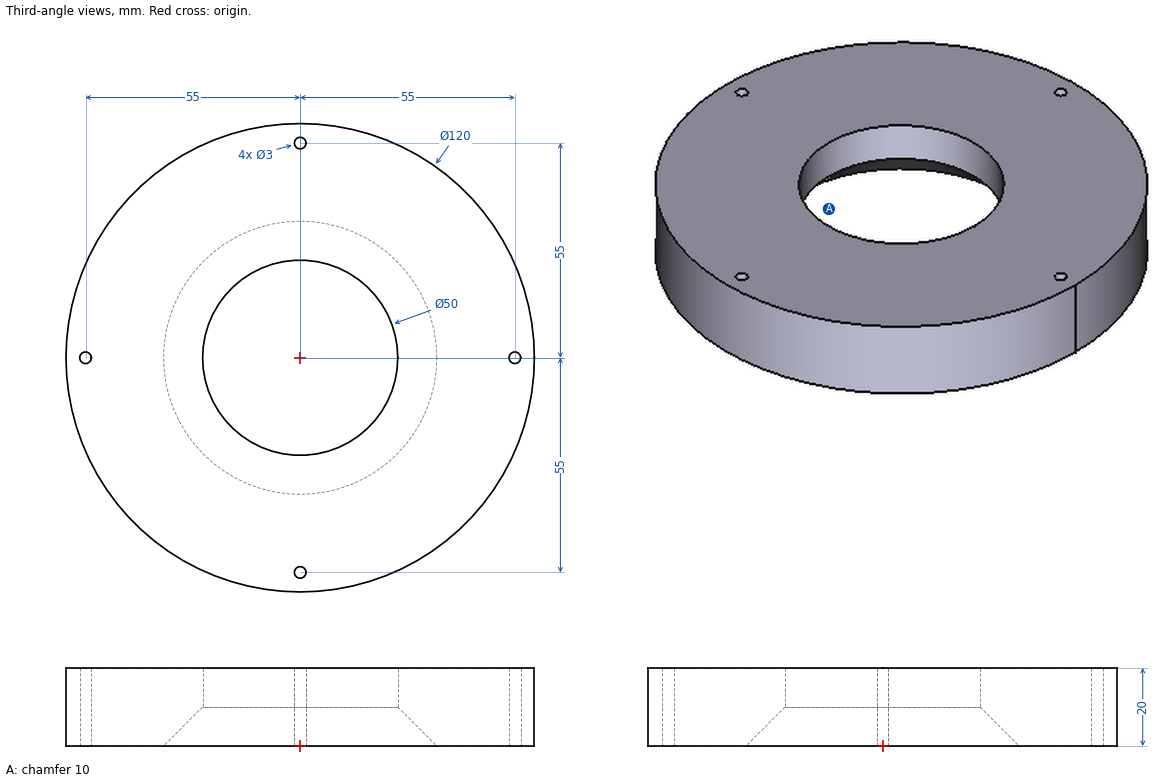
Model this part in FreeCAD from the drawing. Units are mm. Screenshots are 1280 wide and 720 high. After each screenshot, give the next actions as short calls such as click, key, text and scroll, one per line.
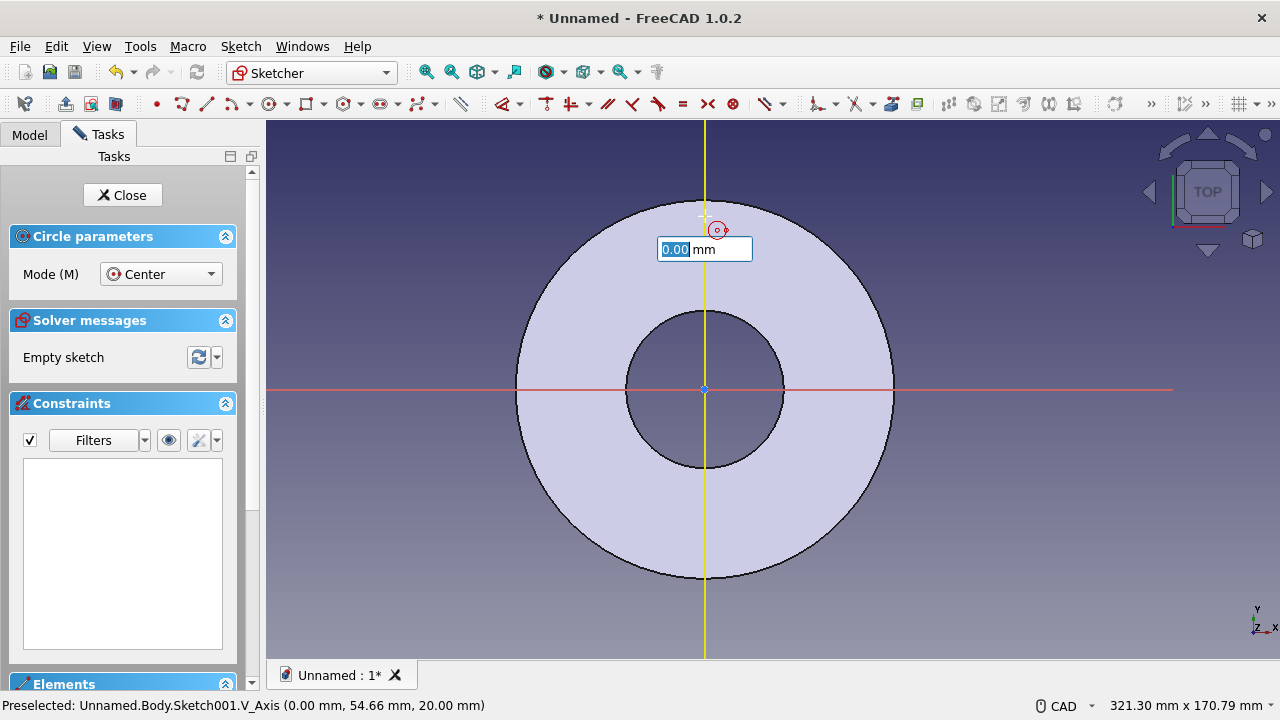
scroll(709, 214, up, 7)
move(709, 215)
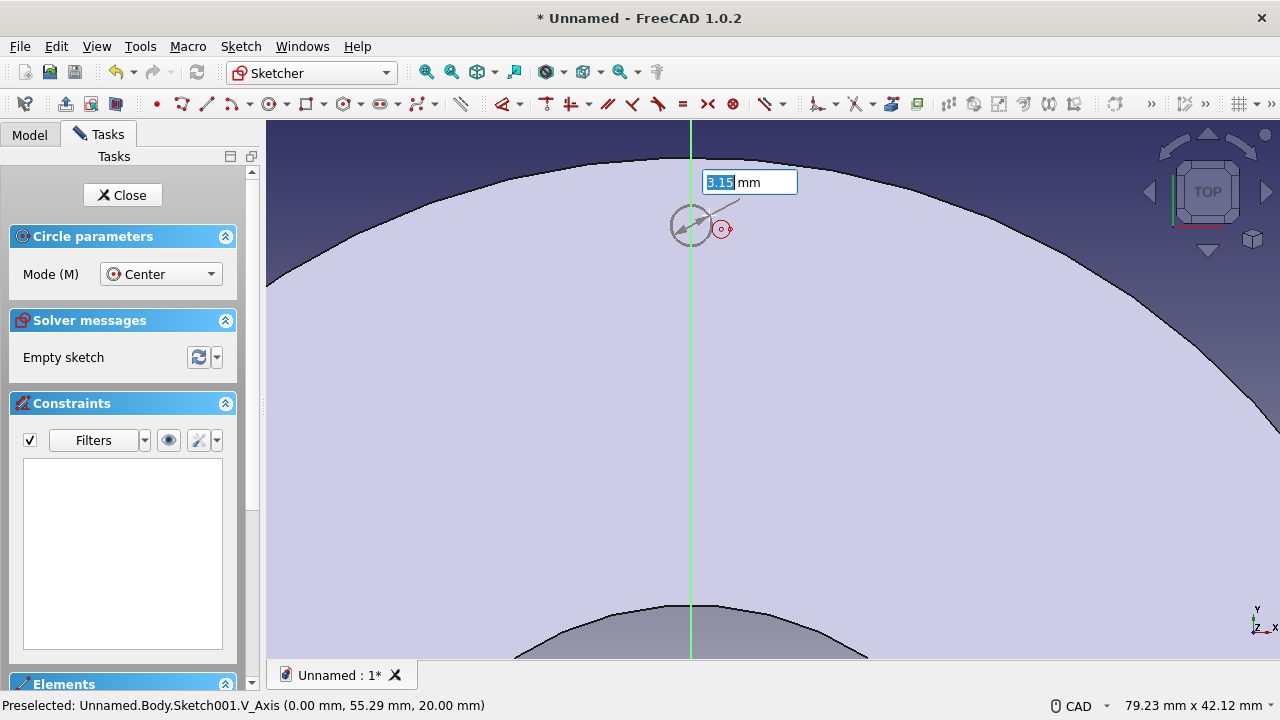
text(3)
key(Return)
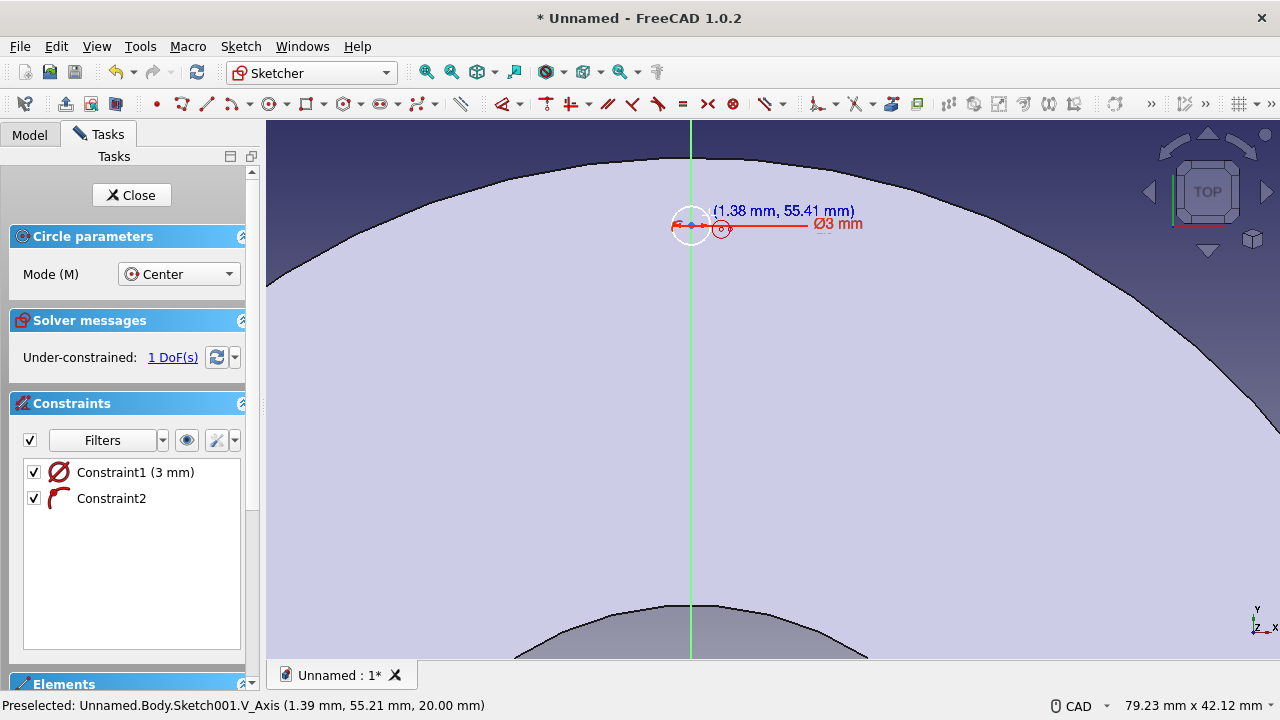
scroll(709, 214, down, 7)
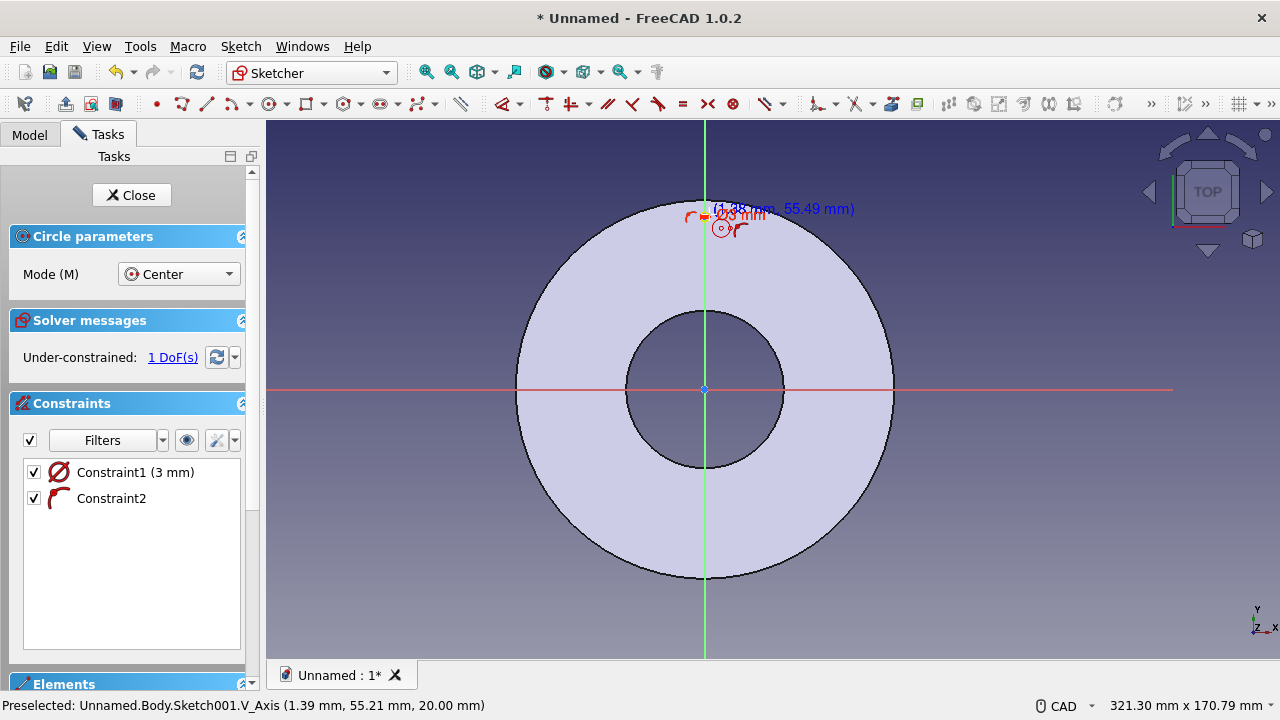
scroll(879, 389, up, 8)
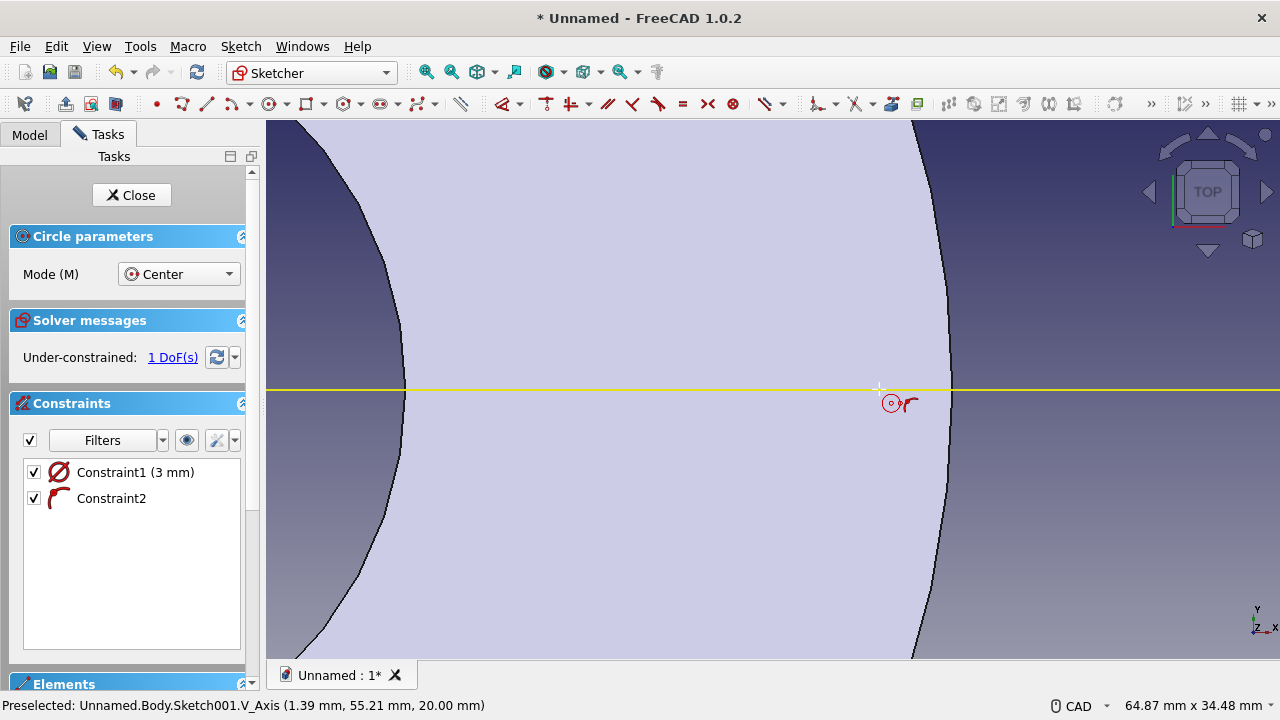
scroll(879, 390, down, 8)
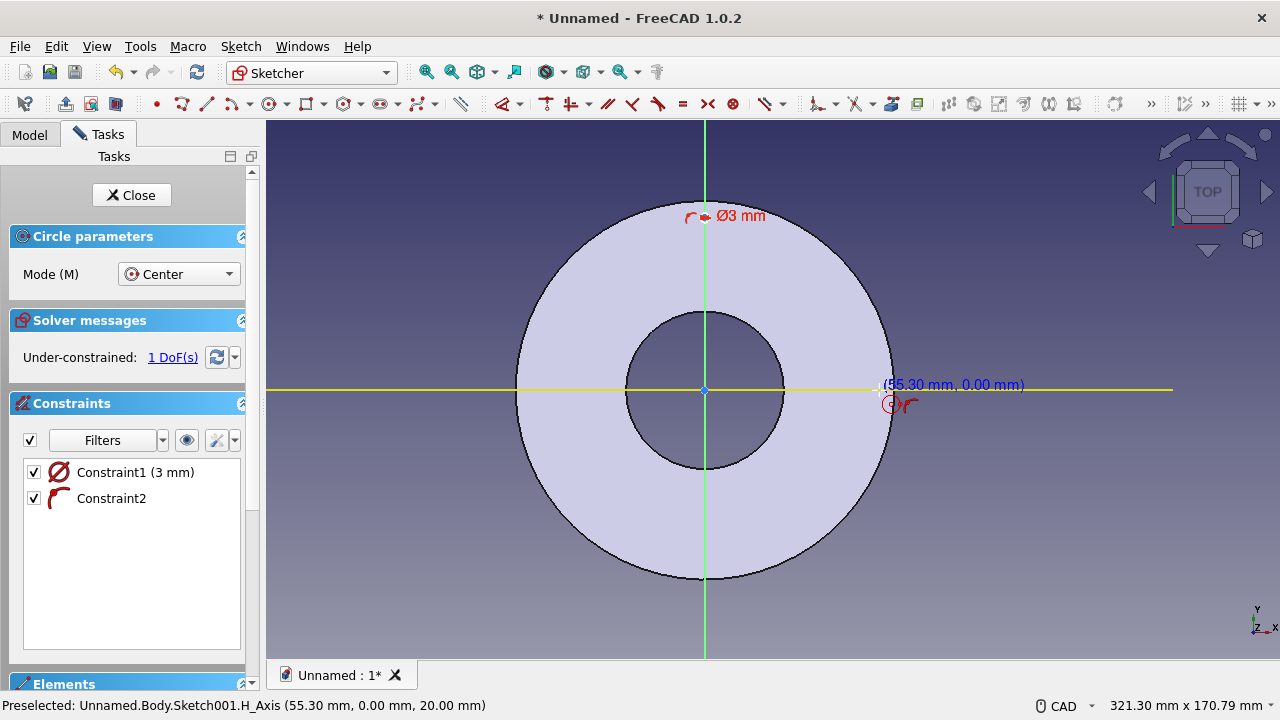
click(879, 390)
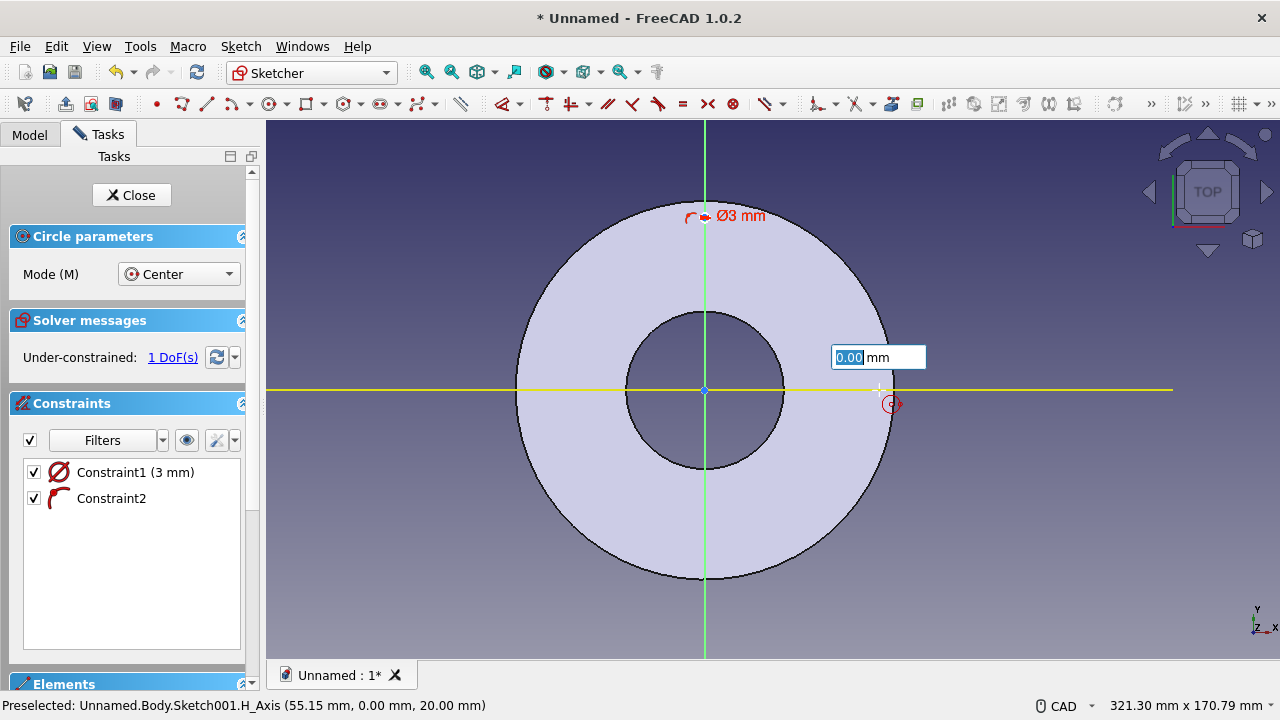
scroll(877, 395, up, 7)
move(875, 392)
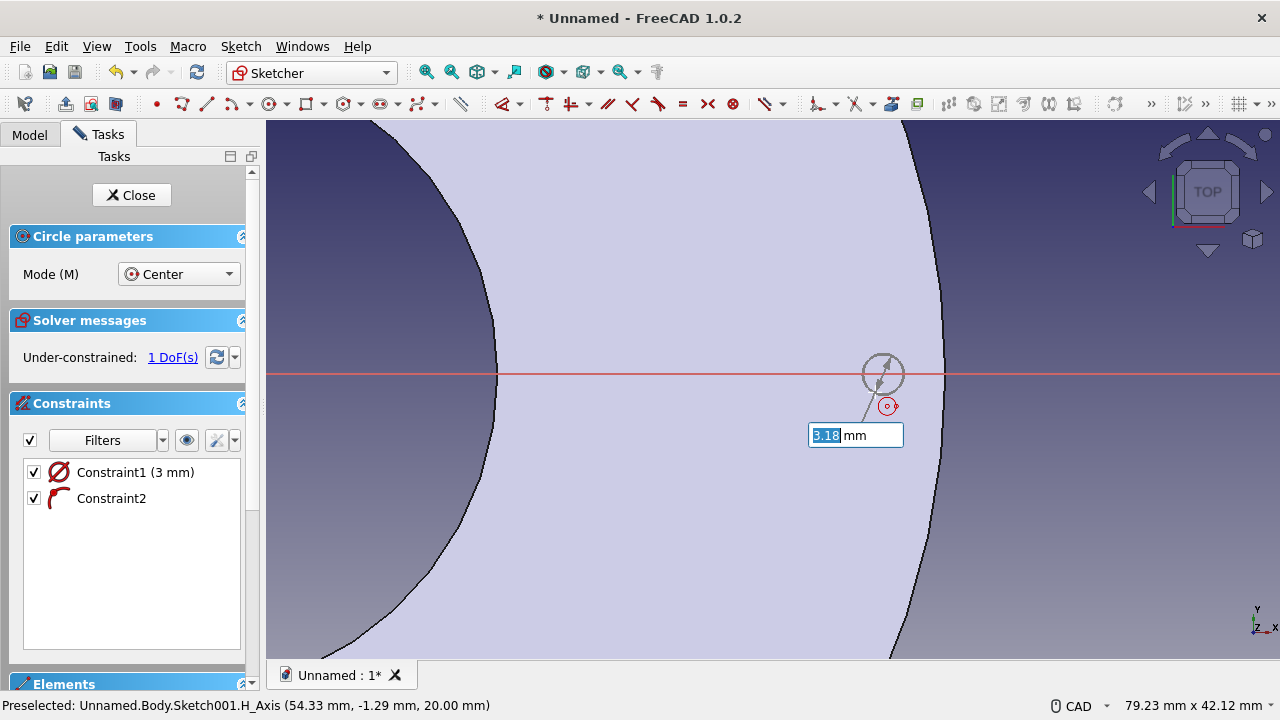
text(3)
key(Return)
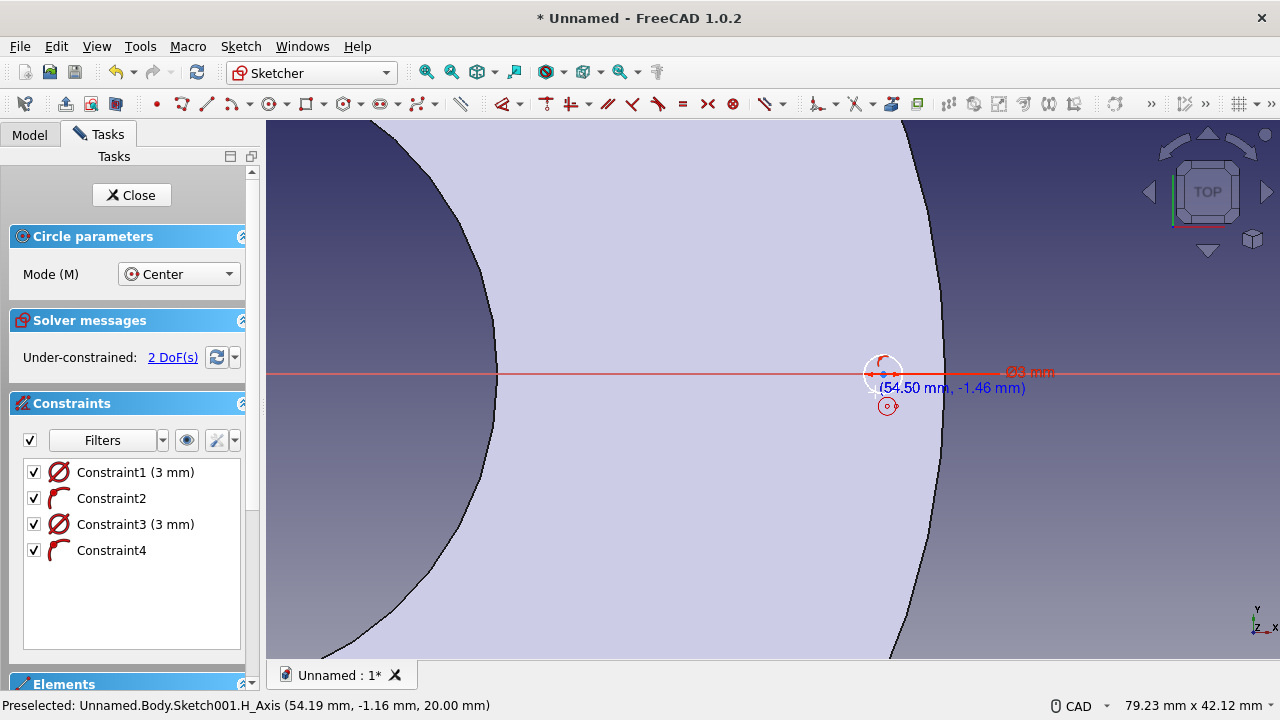
scroll(877, 394, down, 7)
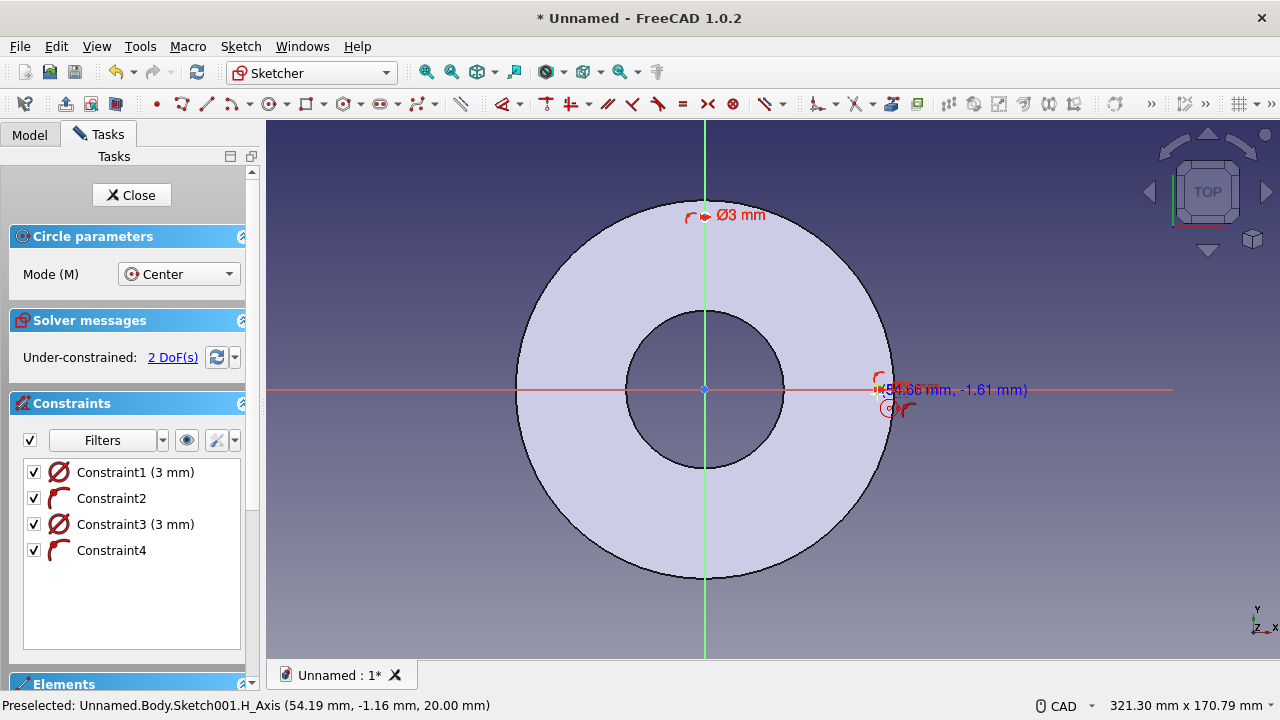
scroll(705, 563, up, 8)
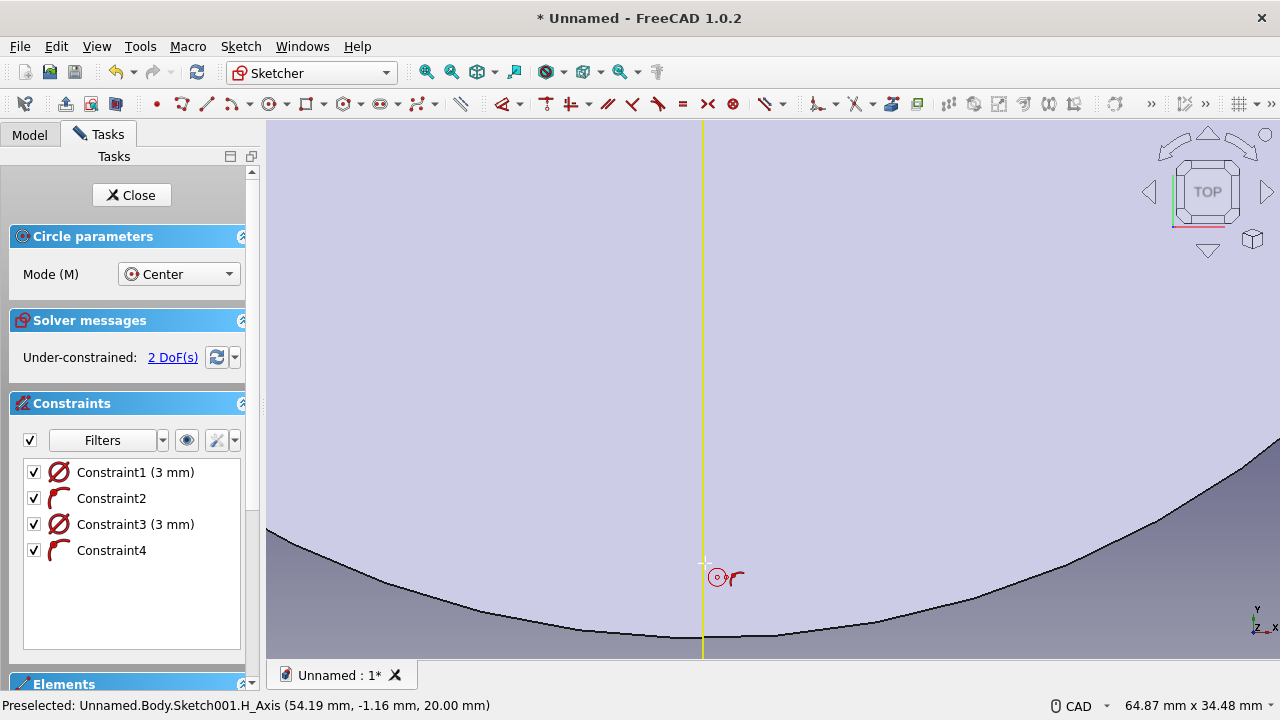
scroll(705, 564, down, 8)